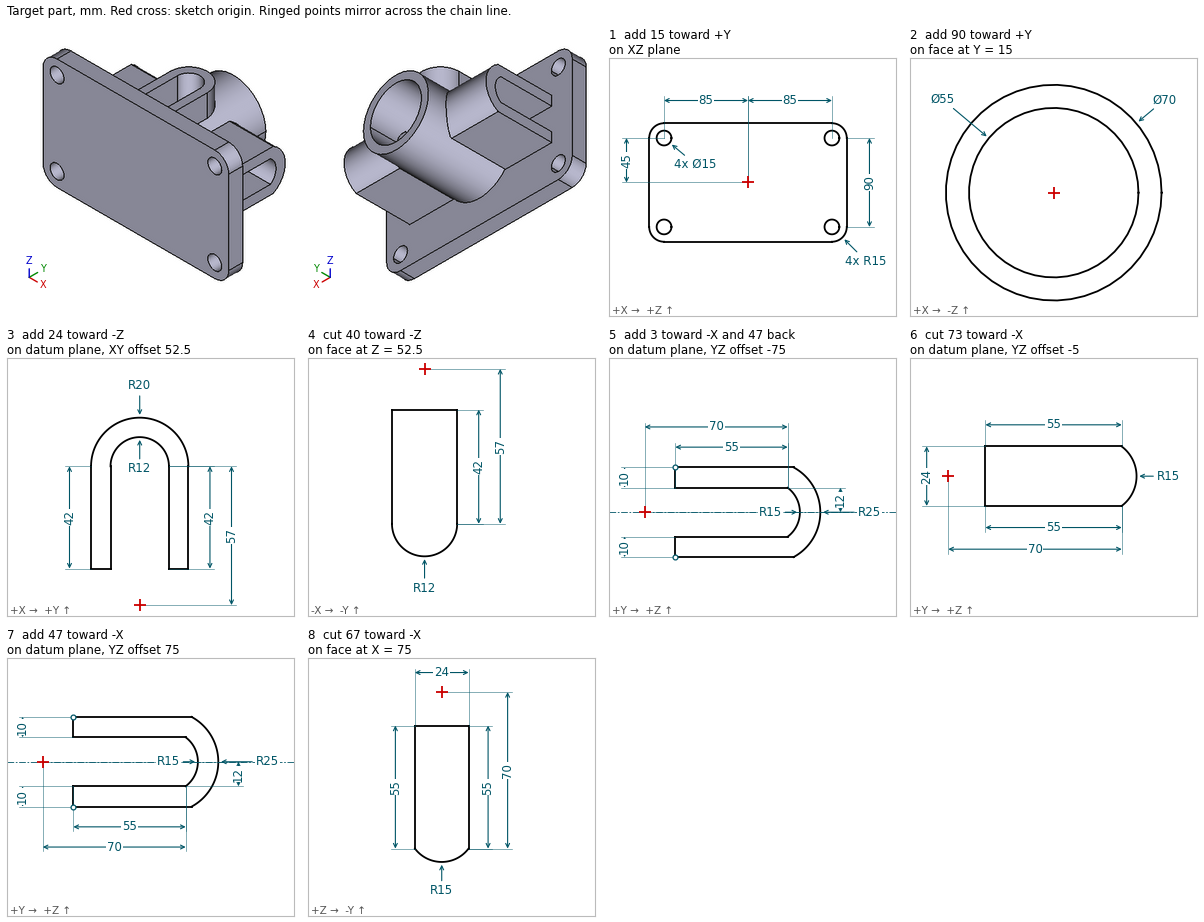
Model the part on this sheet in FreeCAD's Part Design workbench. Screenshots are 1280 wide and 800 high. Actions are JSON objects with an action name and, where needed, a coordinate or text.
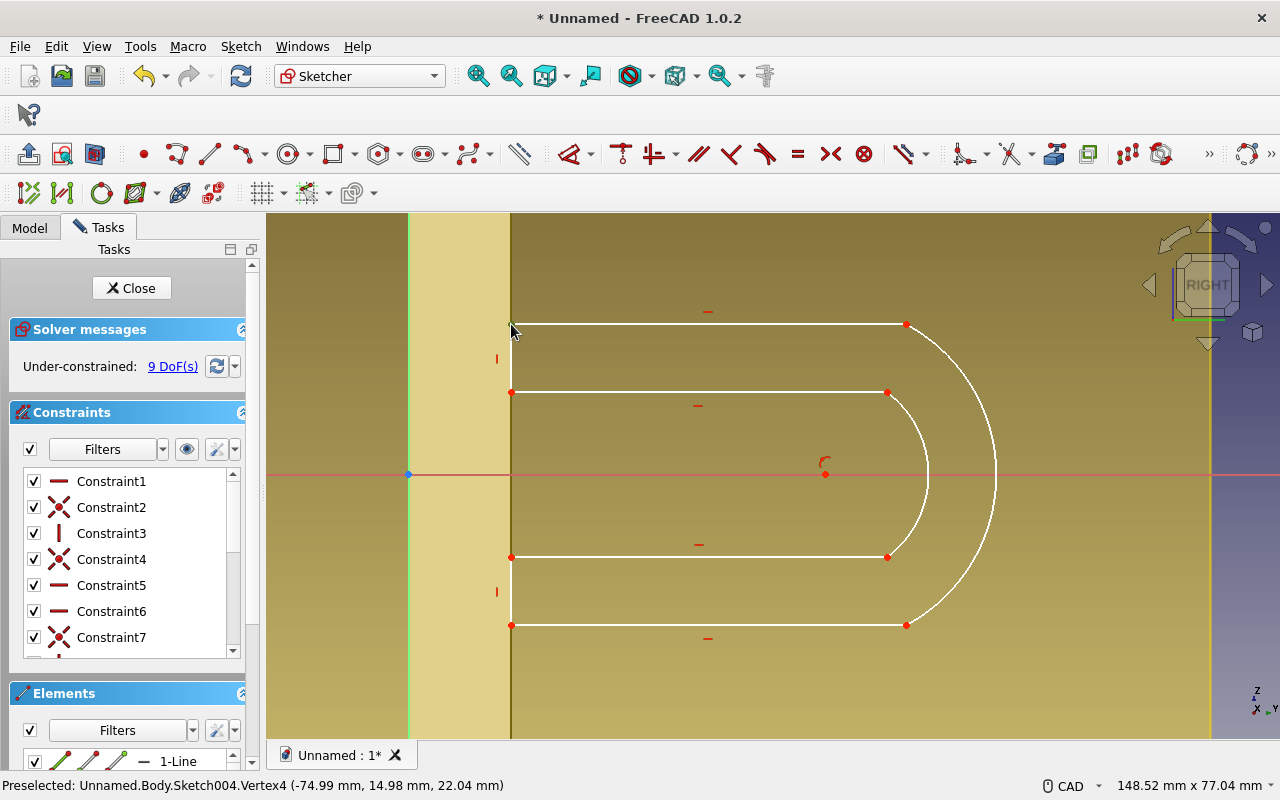
{"action": "left_click", "coordinate": [511, 625]}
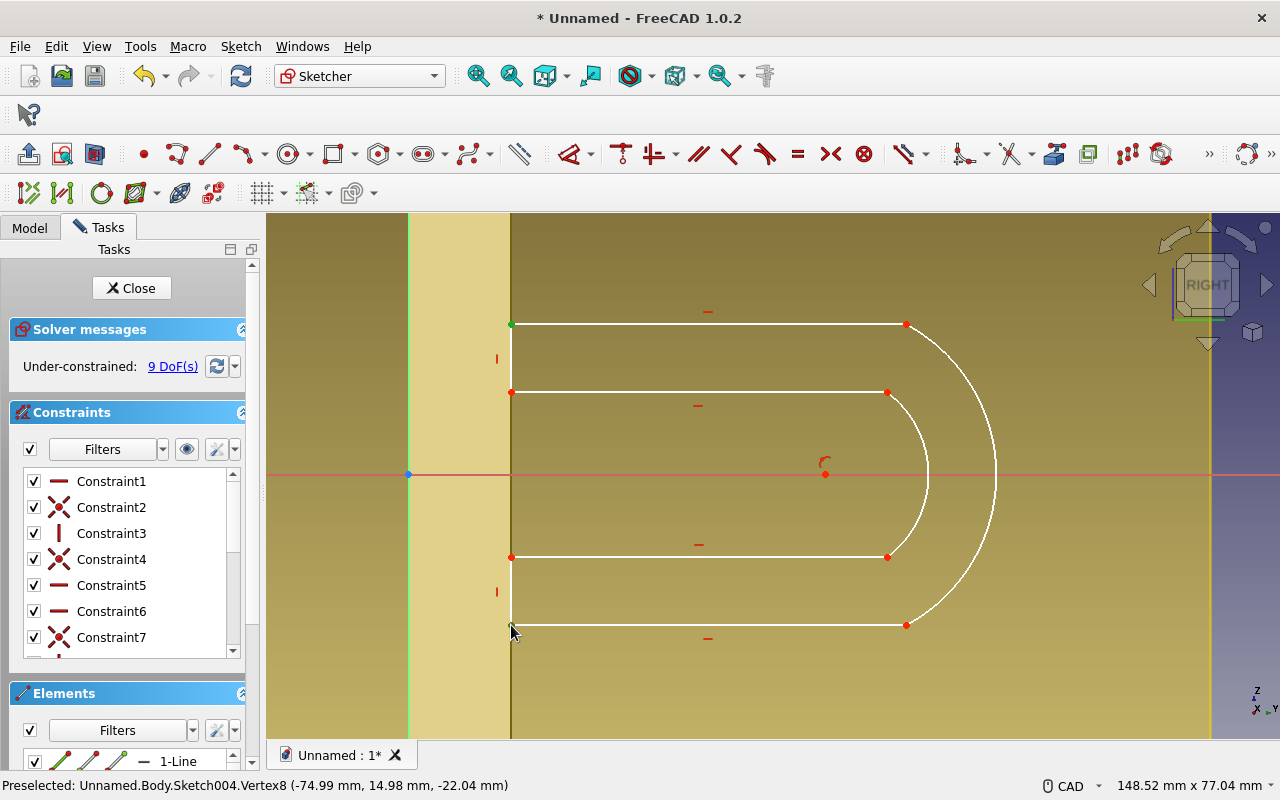
{"action": "left_click", "coordinate": [353, 475]}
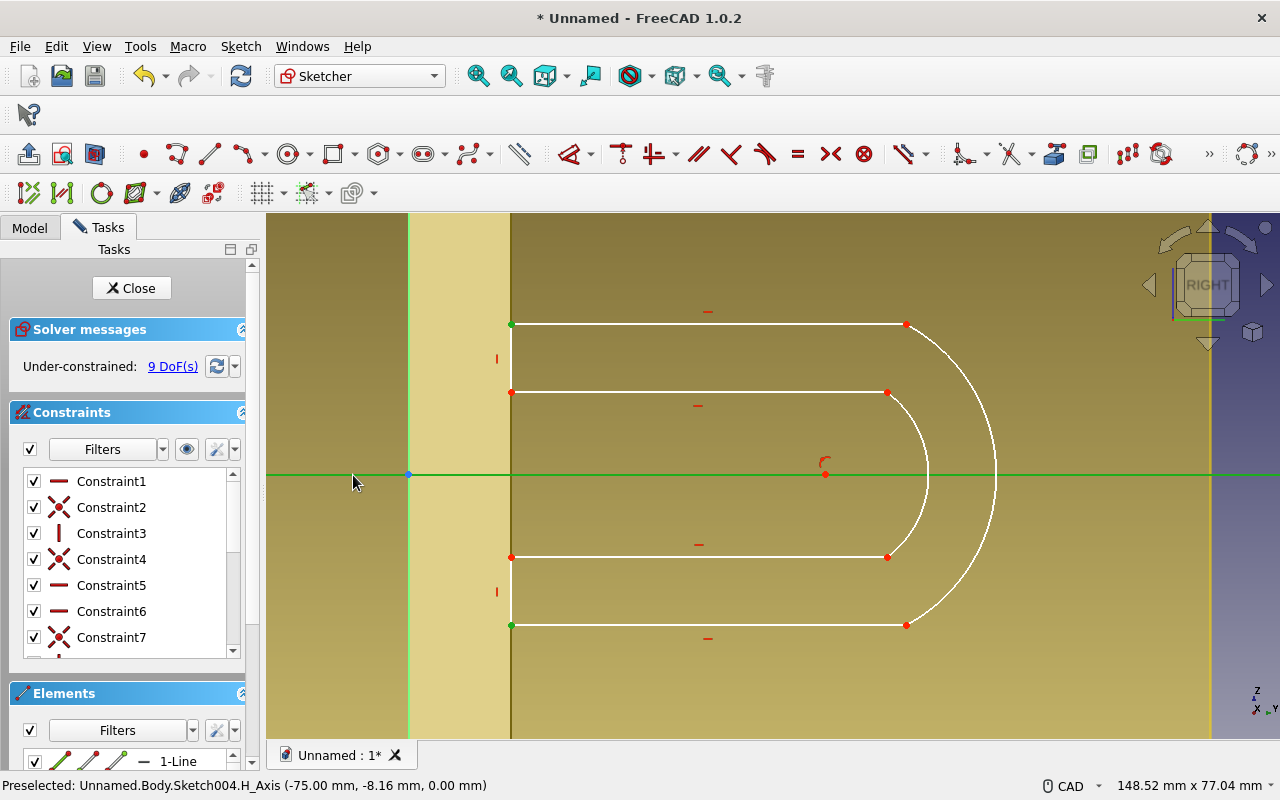
{"action": "key", "text": "s"}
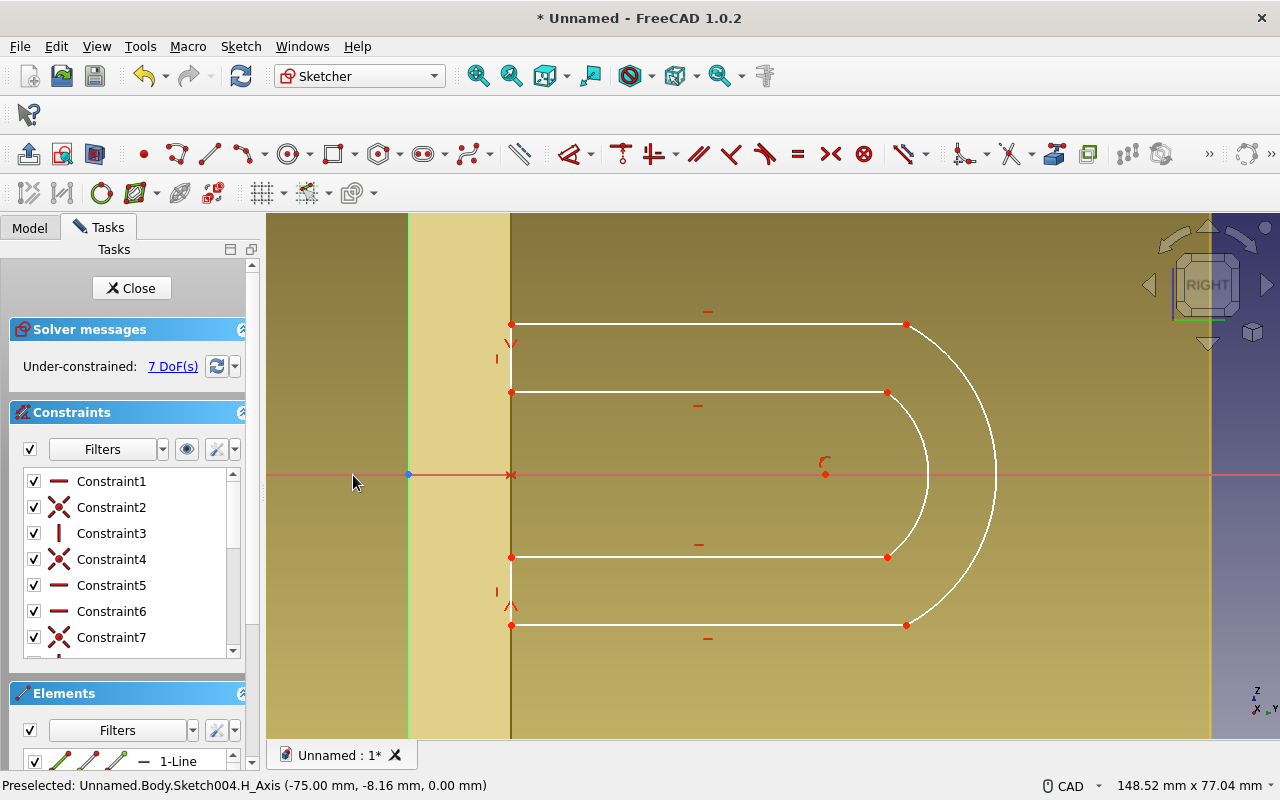
{"action": "left_click", "coordinate": [981, 546]}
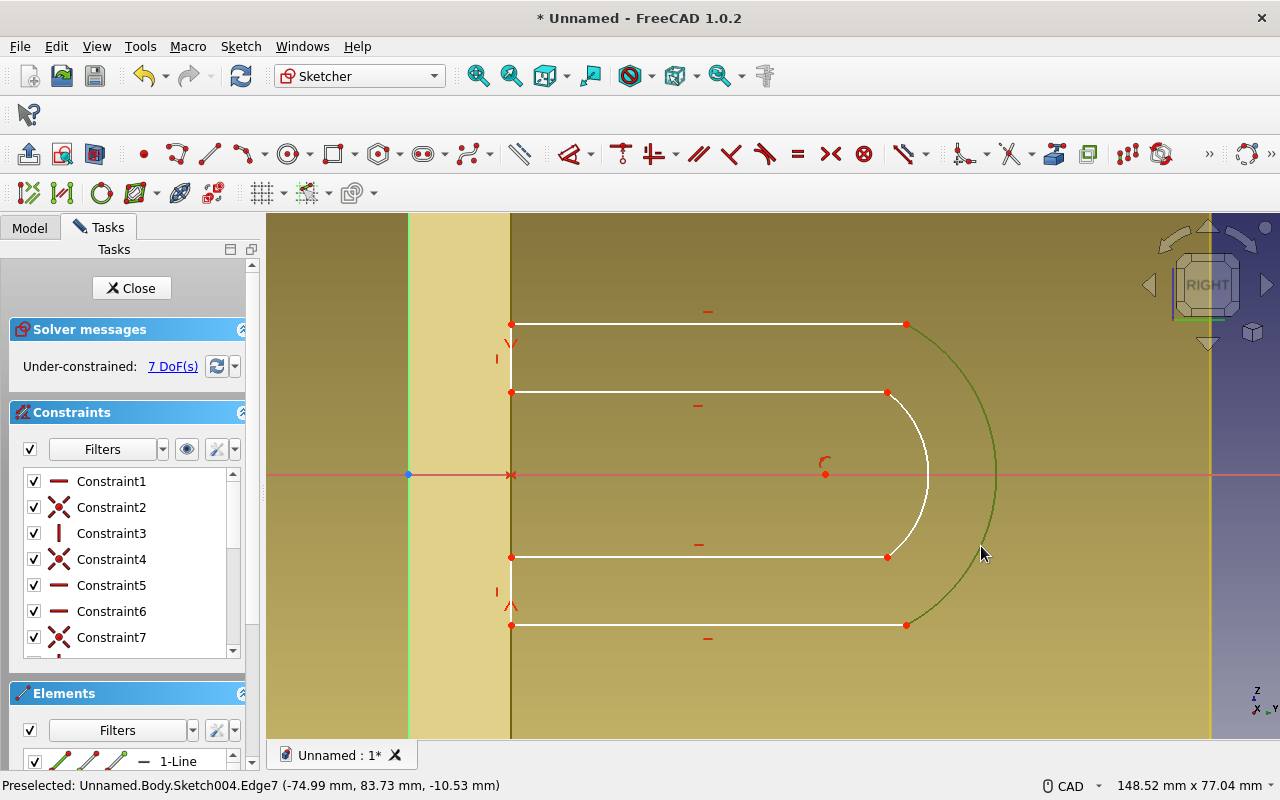
{"action": "left_click", "coordinate": [590, 154]}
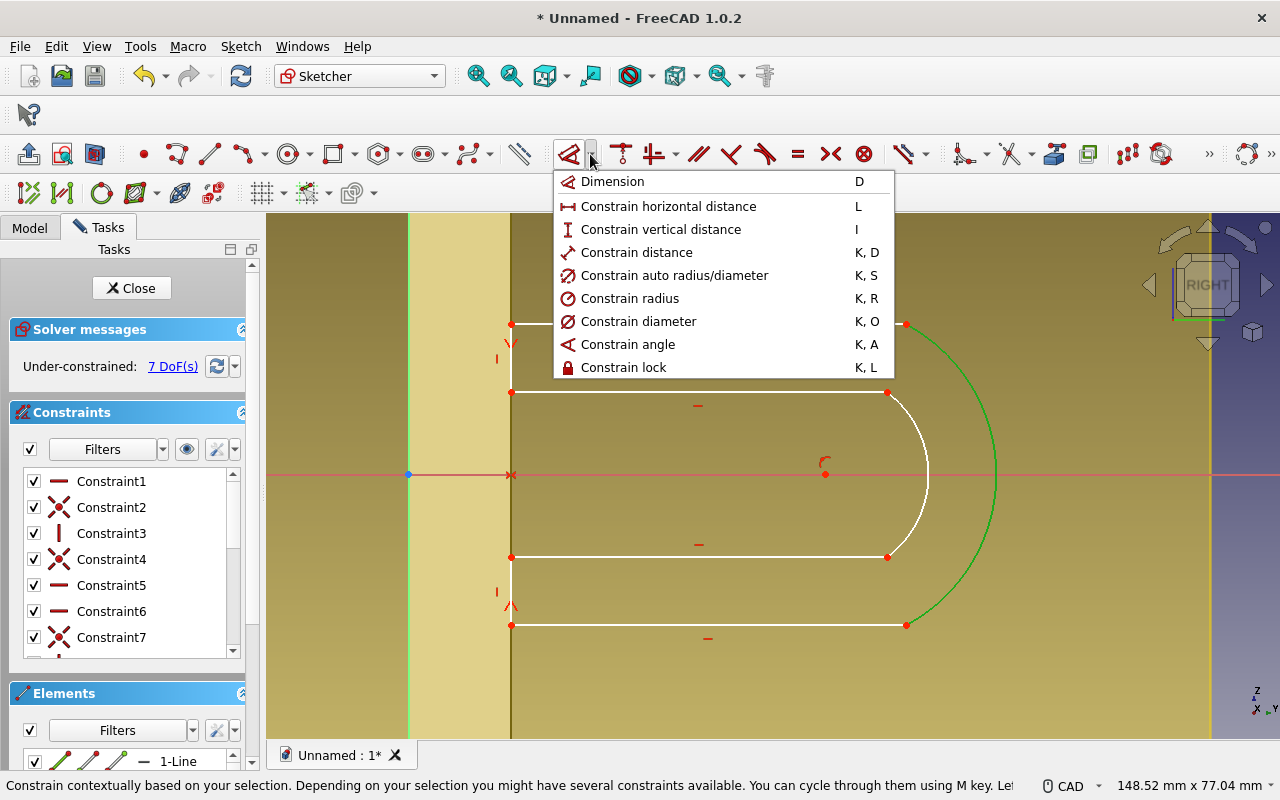
{"action": "left_click", "coordinate": [724, 298]}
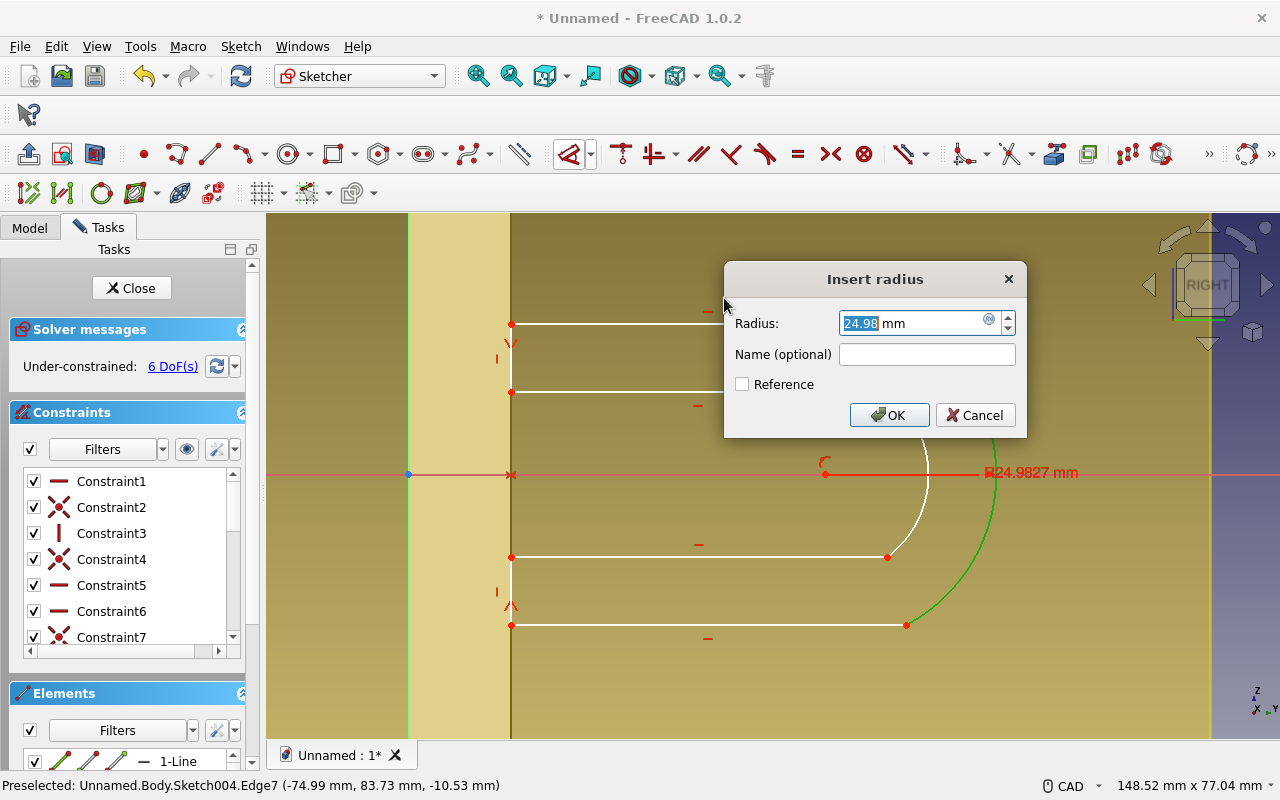
{"action": "type", "text": "25"}
{"action": "key", "text": "Return"}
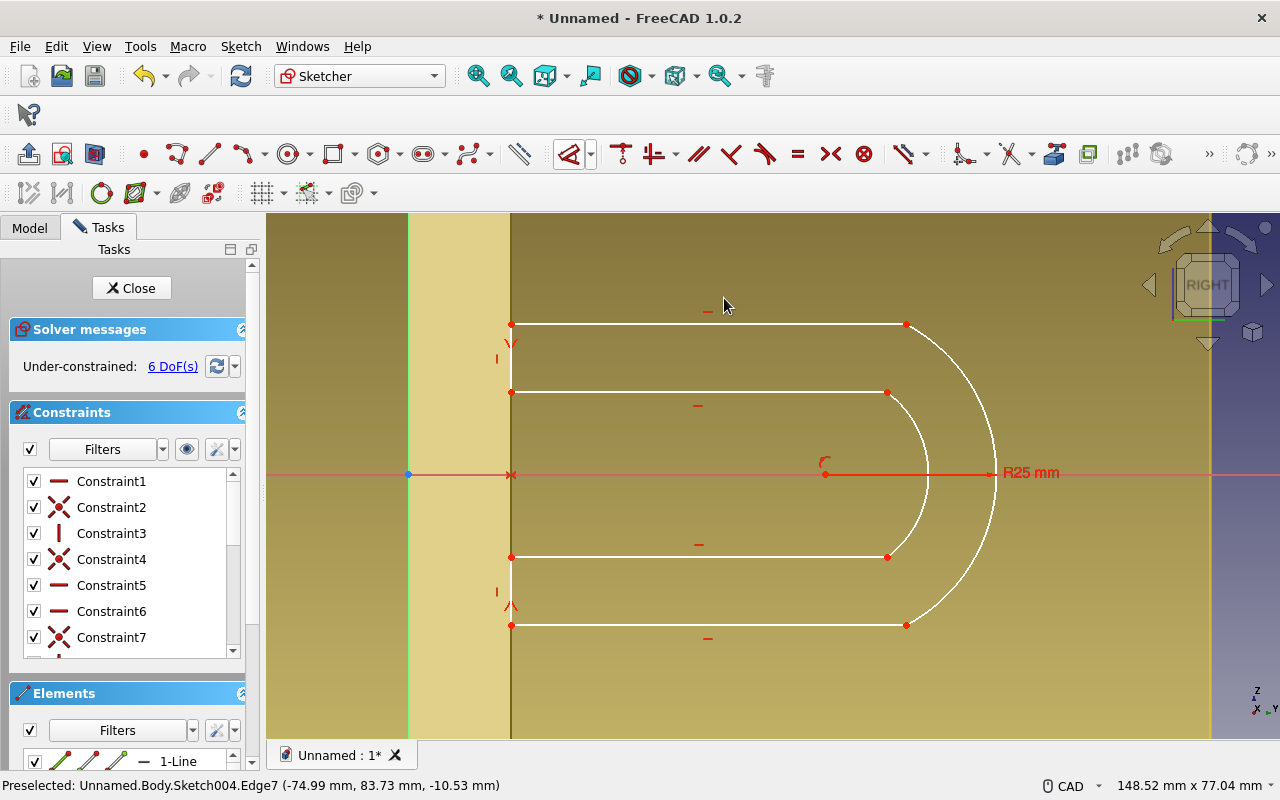
{"action": "left_click", "coordinate": [921, 512]}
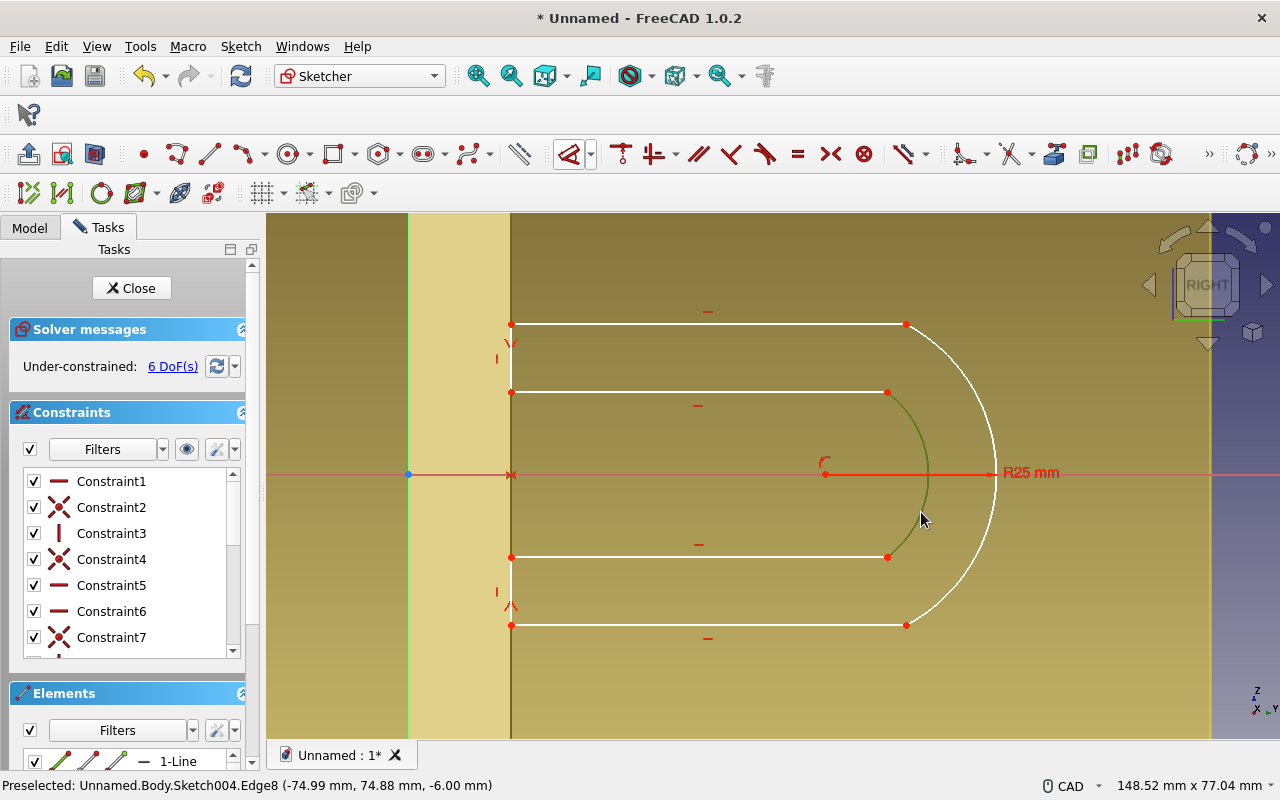
{"action": "key", "text": "k r"}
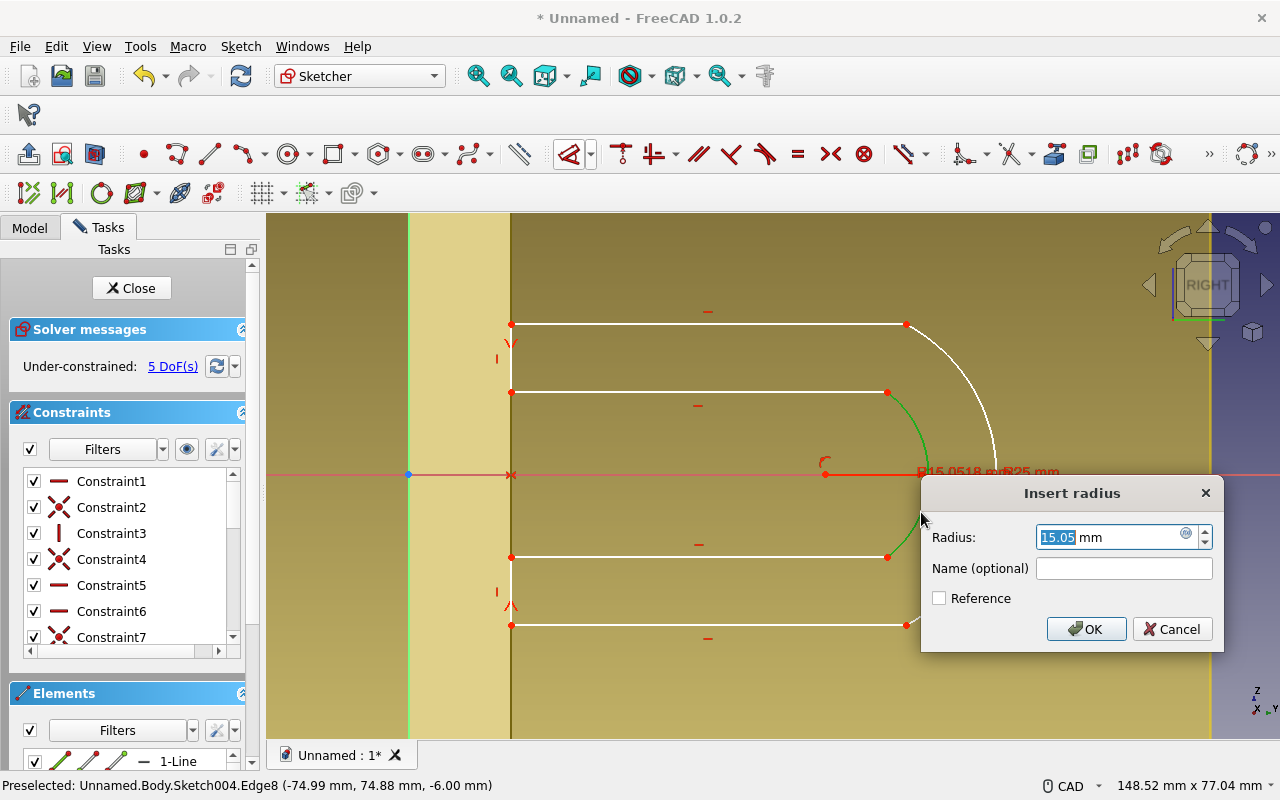
{"action": "type", "text": "15"}
{"action": "key", "text": "Return"}